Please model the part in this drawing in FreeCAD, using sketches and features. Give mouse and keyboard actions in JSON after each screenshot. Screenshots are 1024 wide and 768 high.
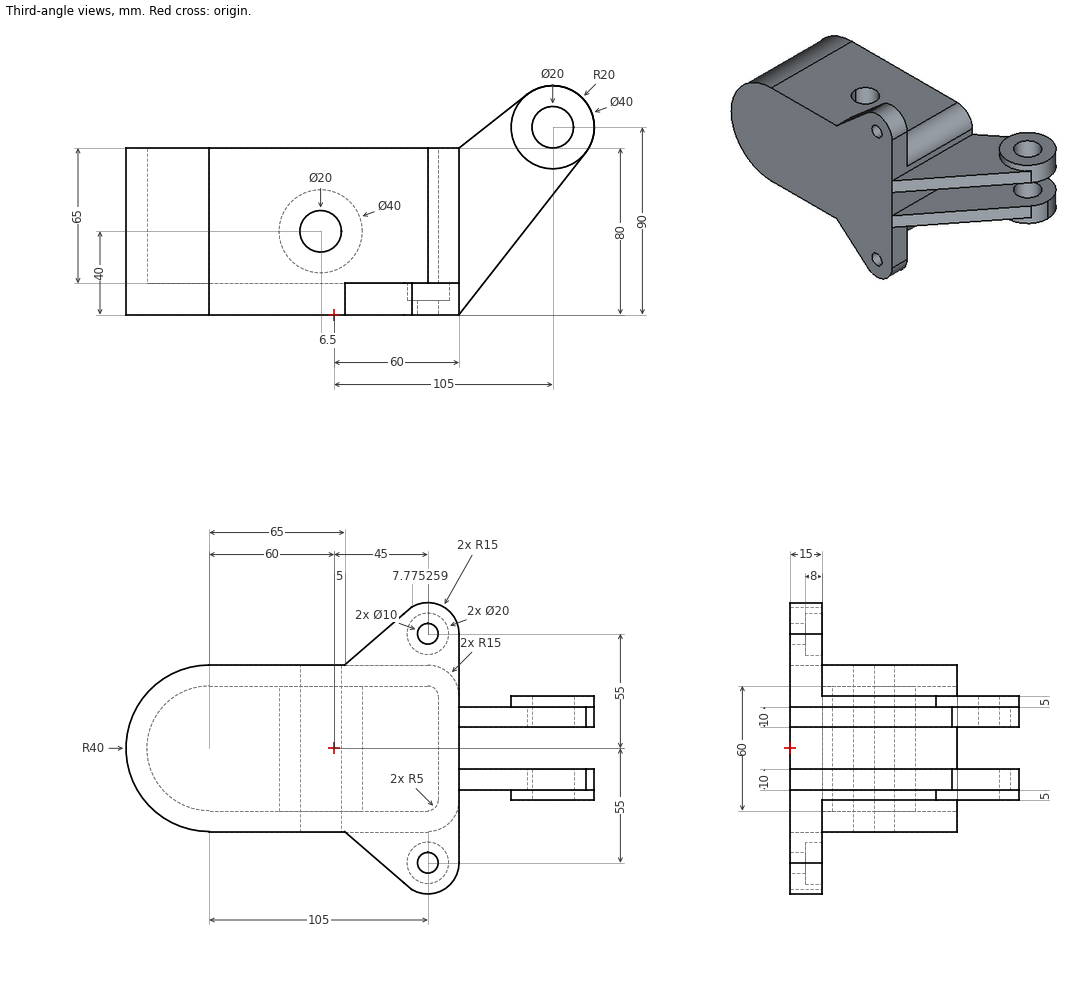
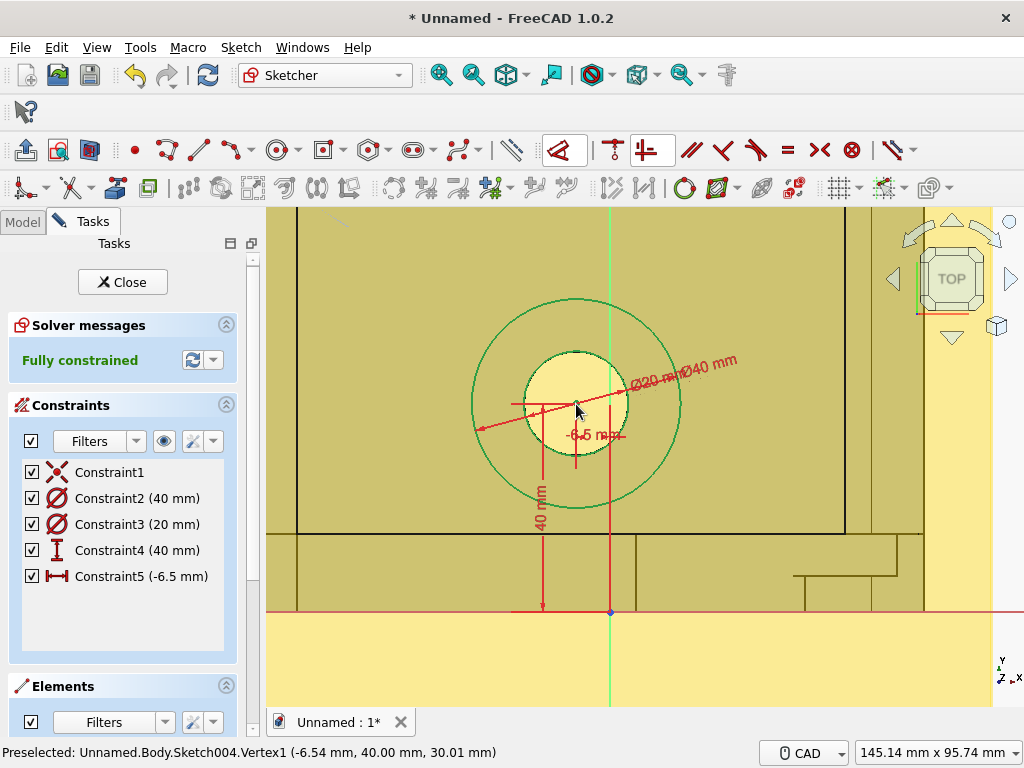
{"action": "left_click", "coordinate": [123, 282]}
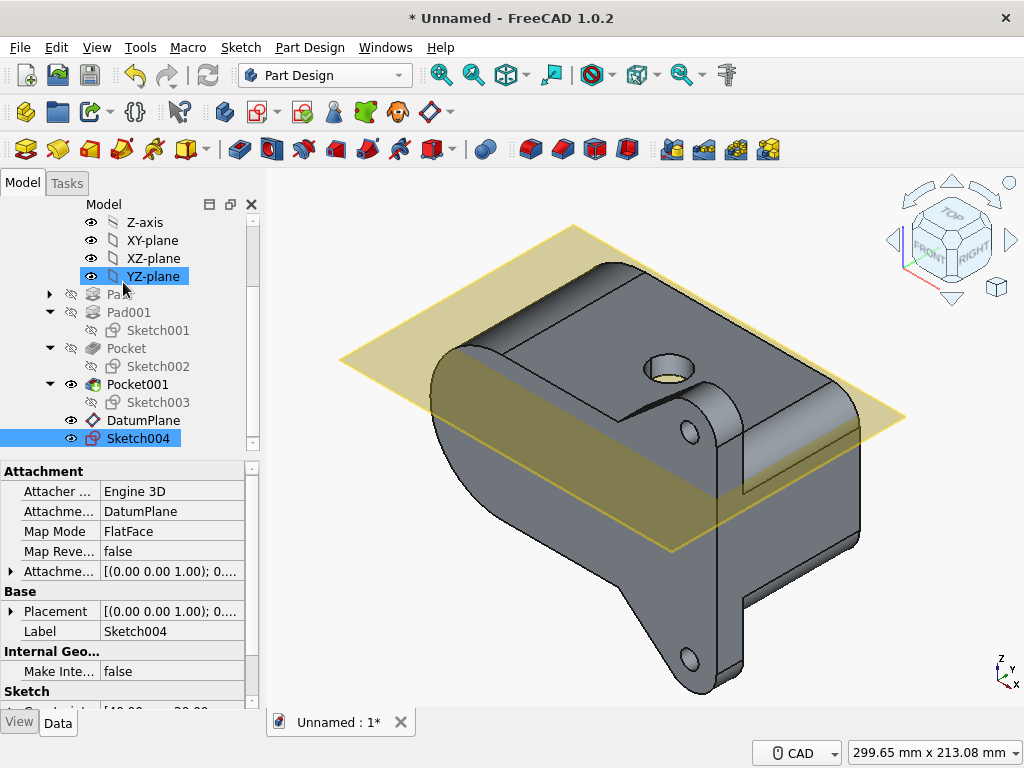
{"action": "left_click", "coordinate": [26, 150]}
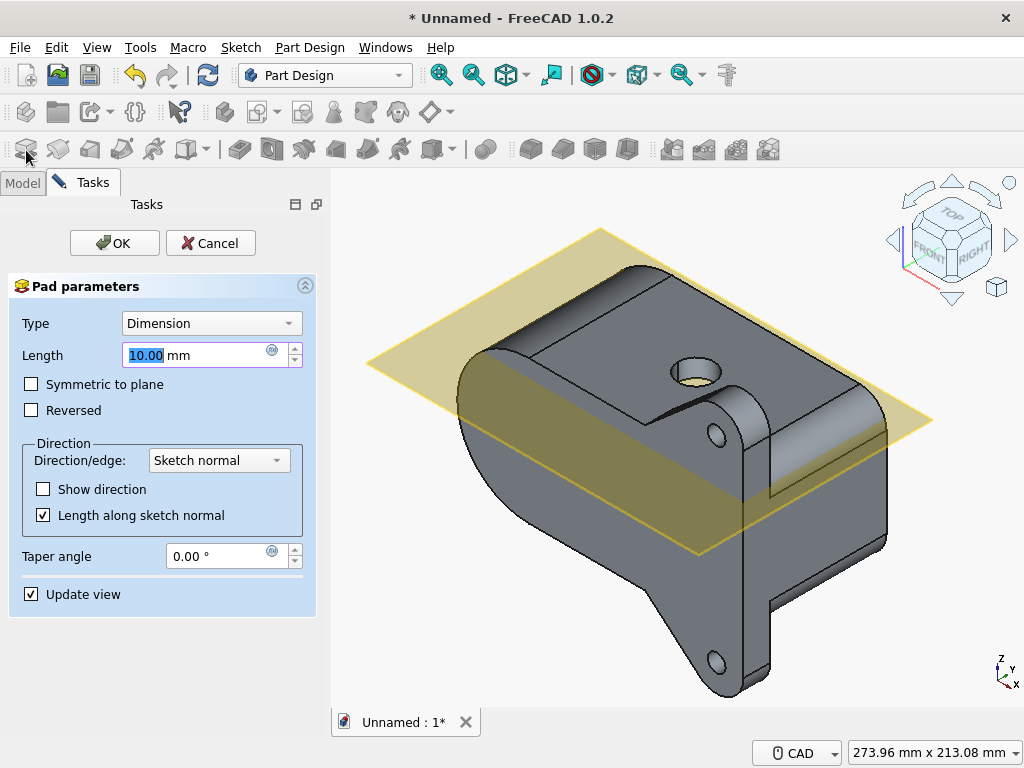
{"action": "type", "text": "60"}
{"action": "key", "text": "Tab"}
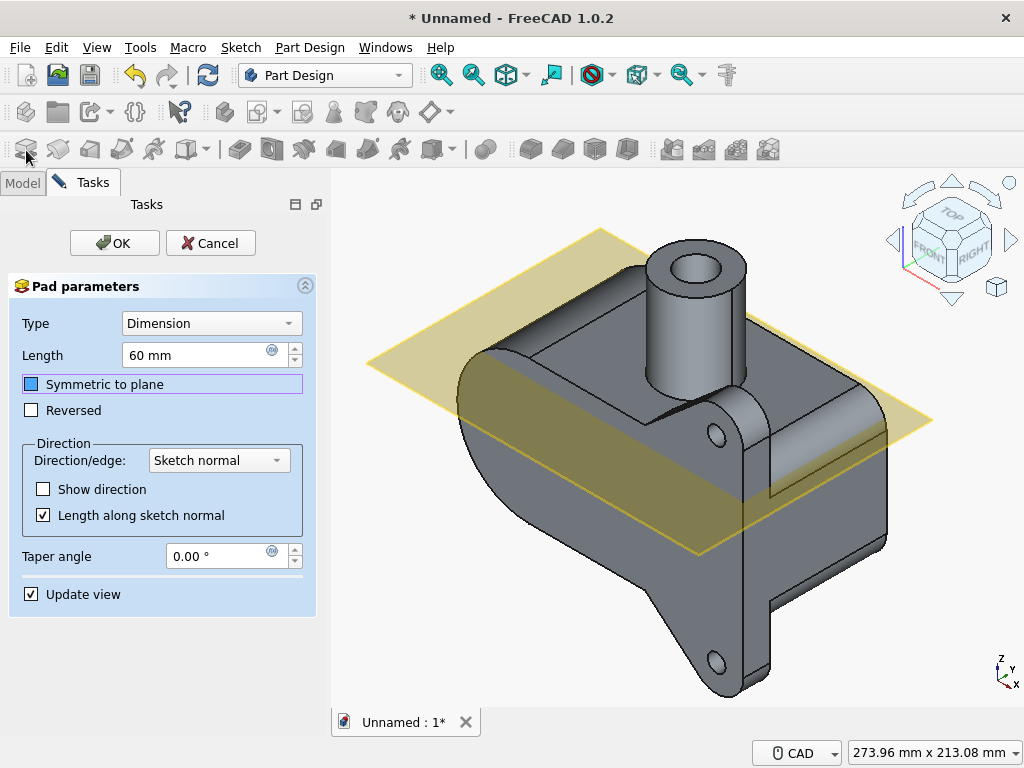
{"action": "left_click", "coordinate": [30, 410]}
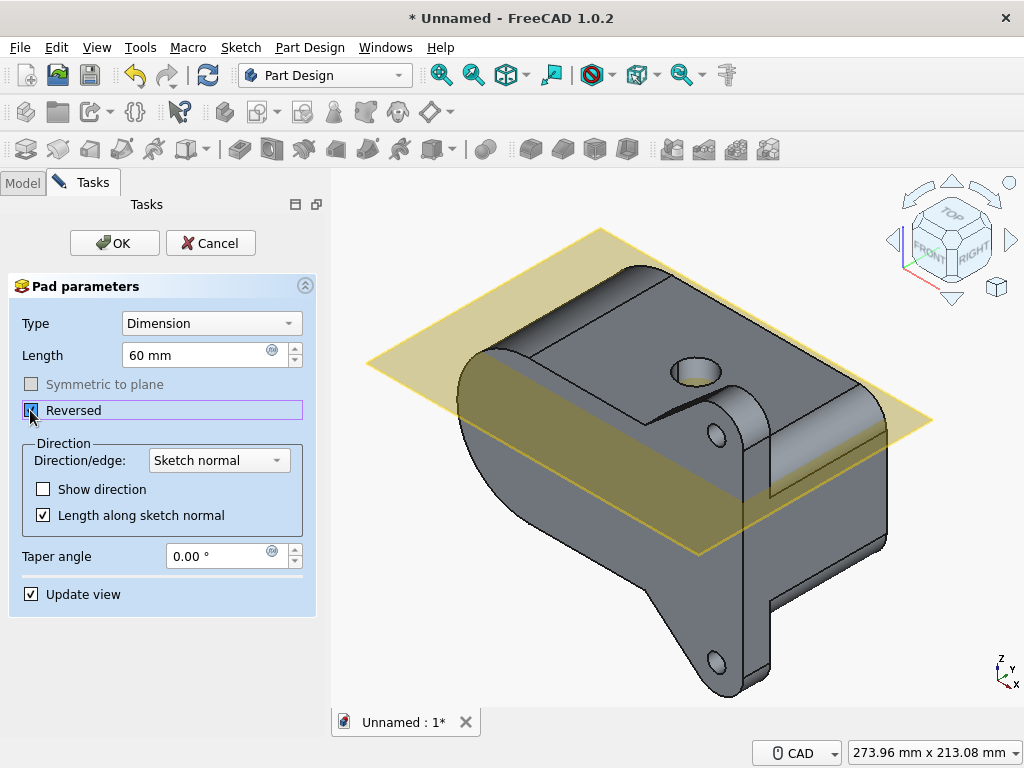
{"action": "left_click", "coordinate": [115, 243]}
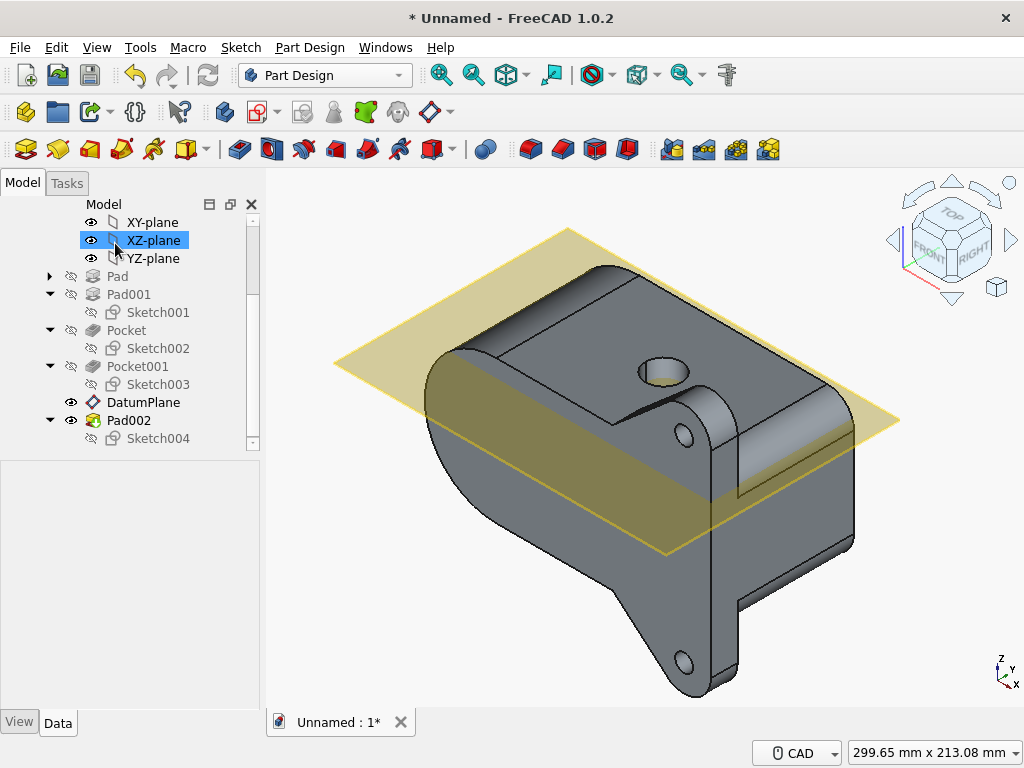
{"action": "left_click", "coordinate": [116, 402]}
{"action": "key", "text": "space"}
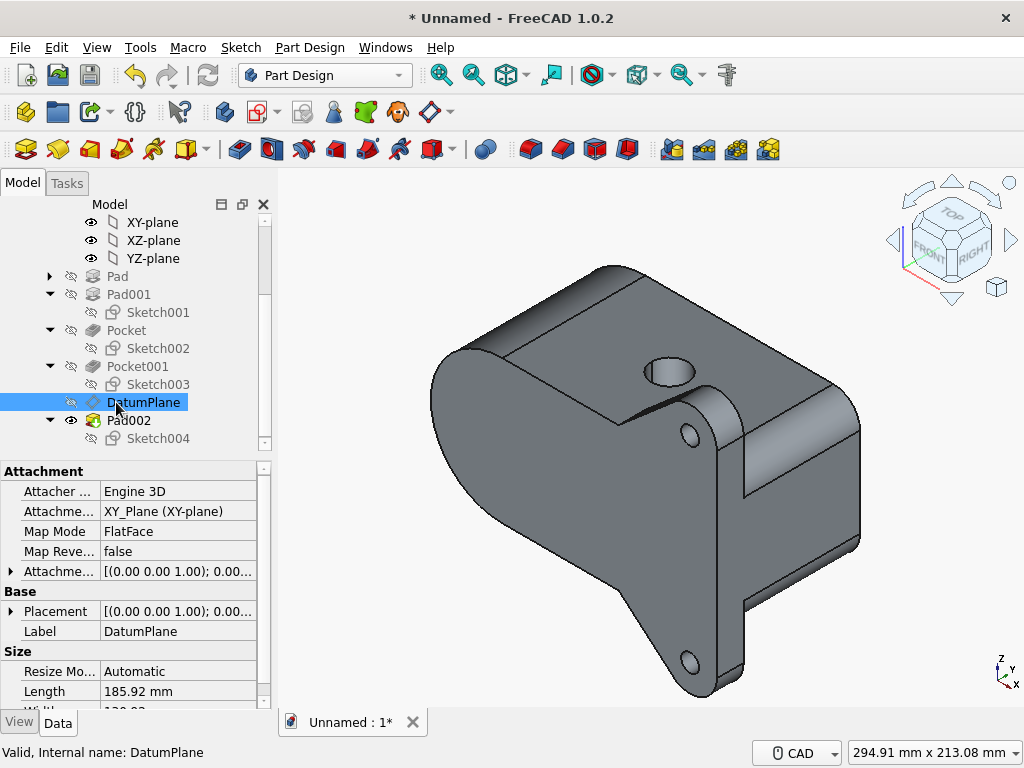
{"action": "left_click", "coordinate": [442, 76]}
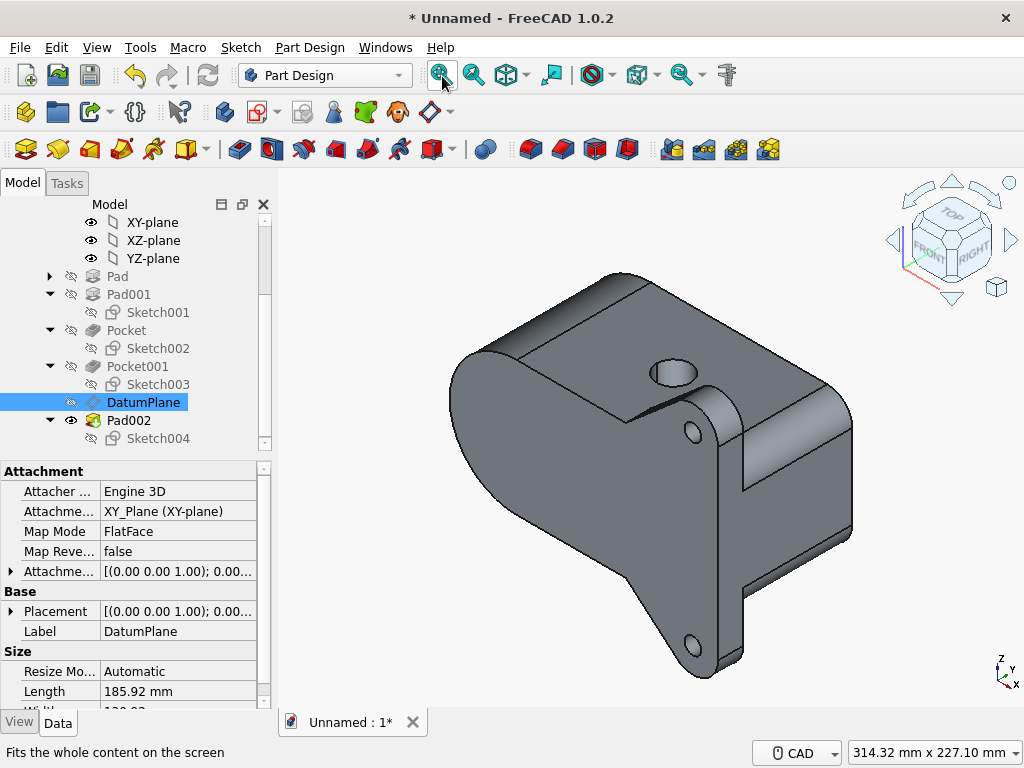
{"action": "scroll", "coordinate": [160, 326], "scroll_direction": "down", "scroll_amount": 3}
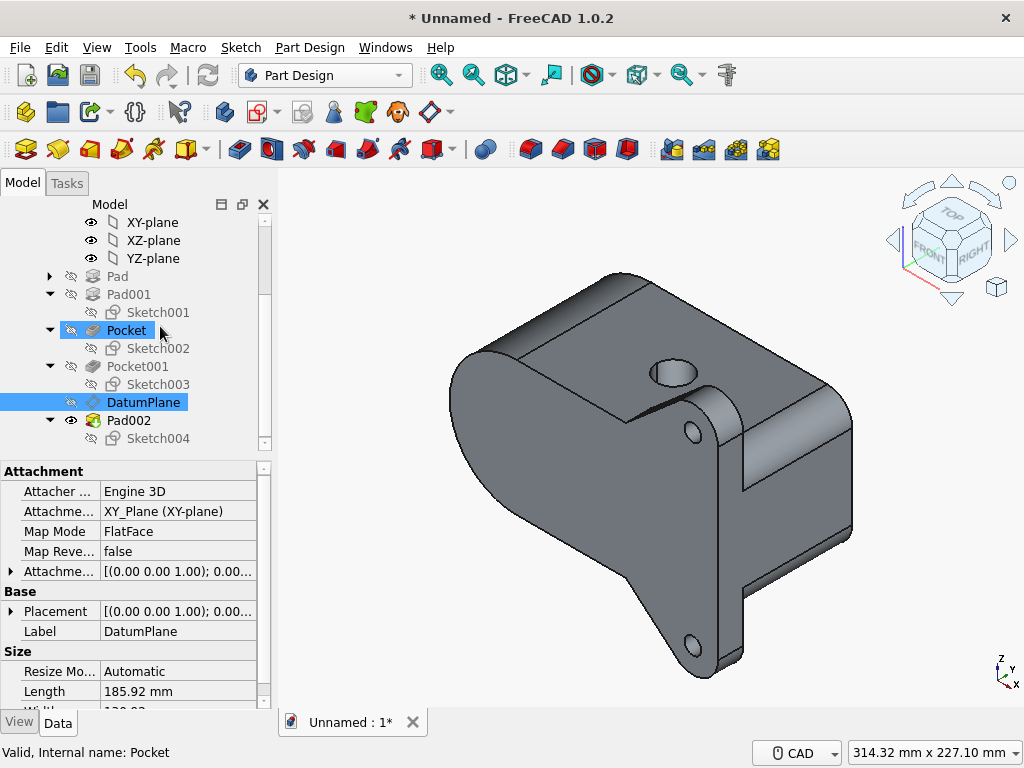
{"action": "scroll", "coordinate": [160, 326], "scroll_direction": "up", "scroll_amount": 15}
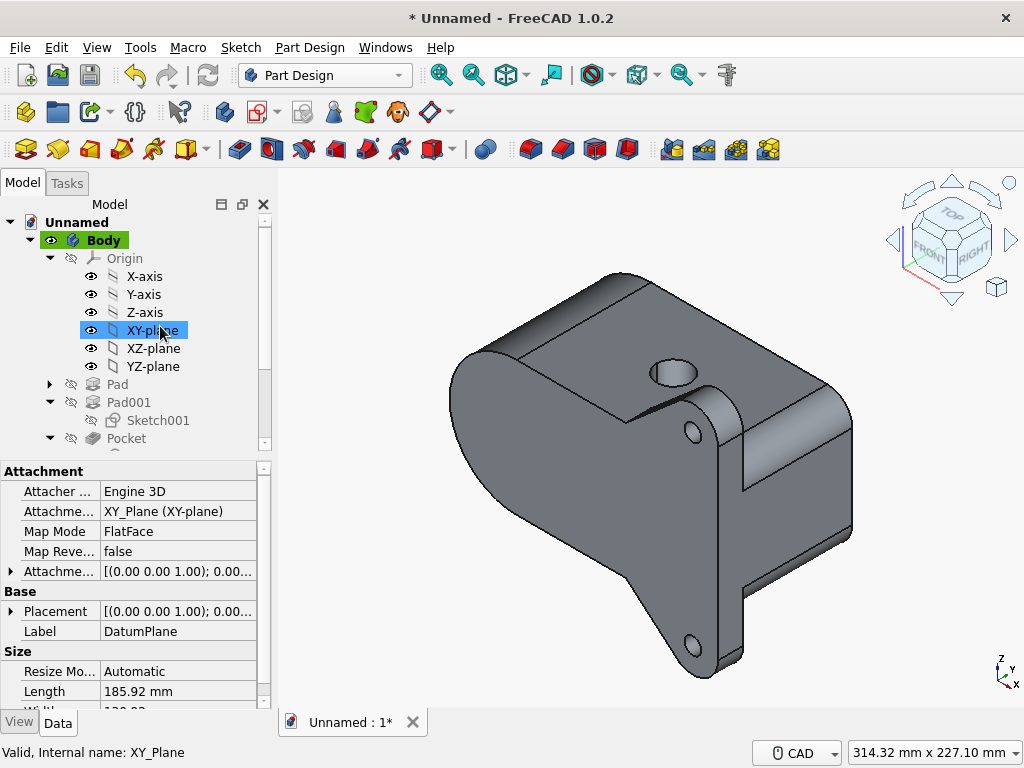
{"action": "left_click", "coordinate": [136, 330]}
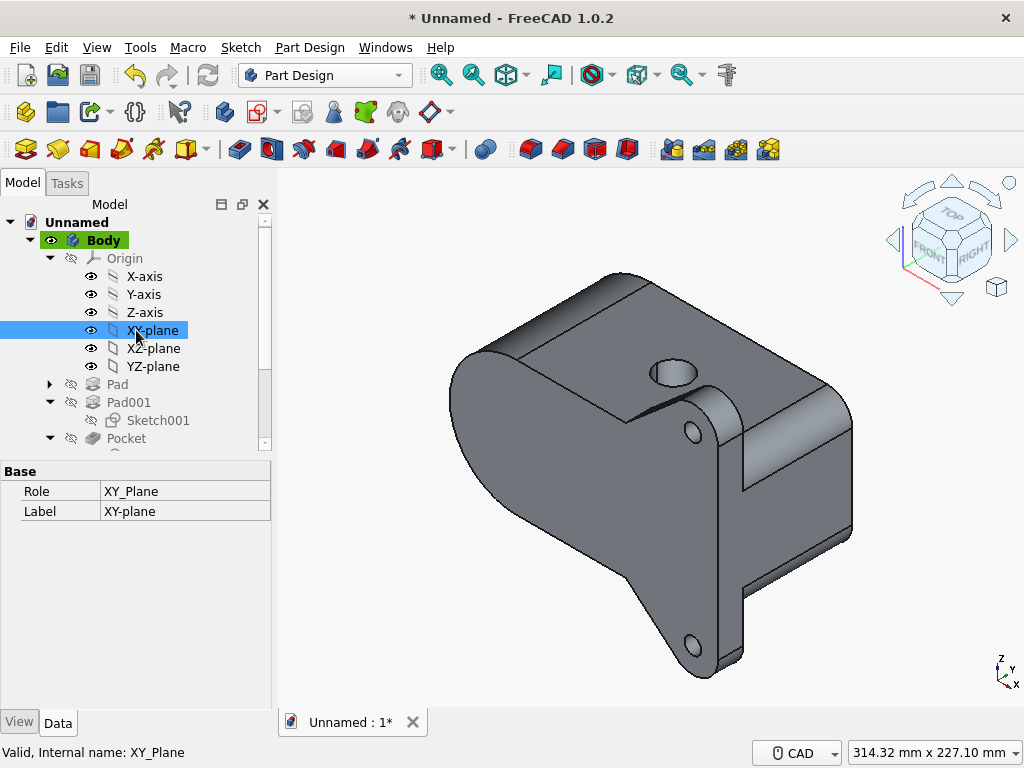
{"action": "left_click", "coordinate": [430, 112]}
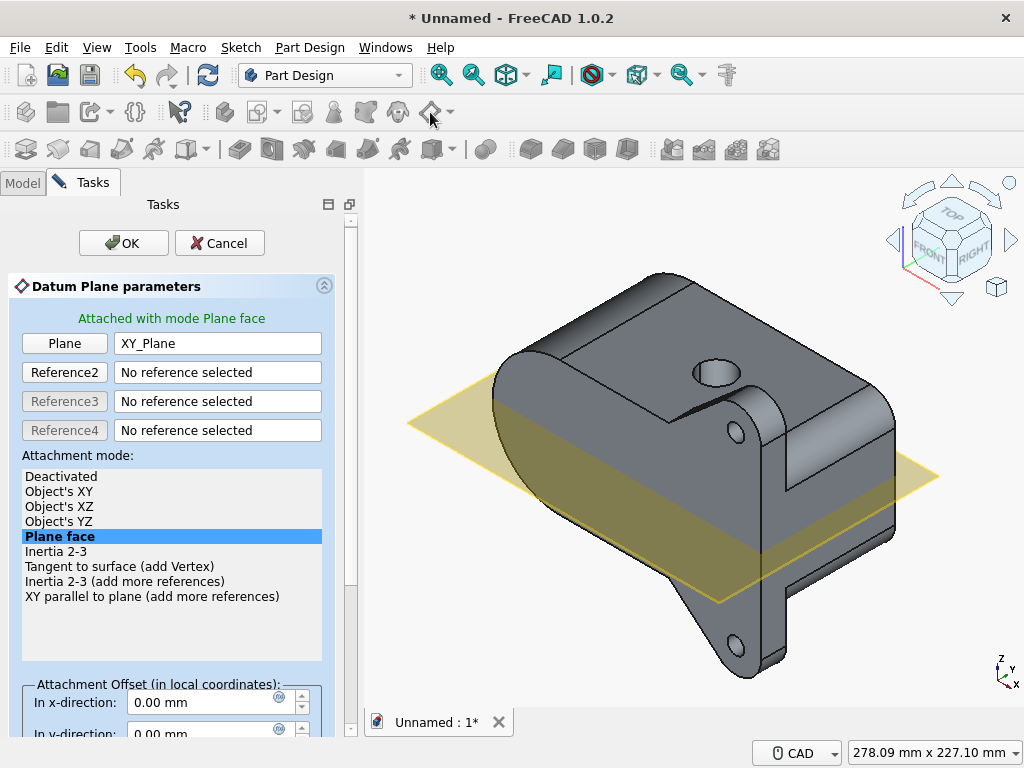
{"action": "scroll", "coordinate": [351, 475], "scroll_direction": "down", "scroll_amount": 2}